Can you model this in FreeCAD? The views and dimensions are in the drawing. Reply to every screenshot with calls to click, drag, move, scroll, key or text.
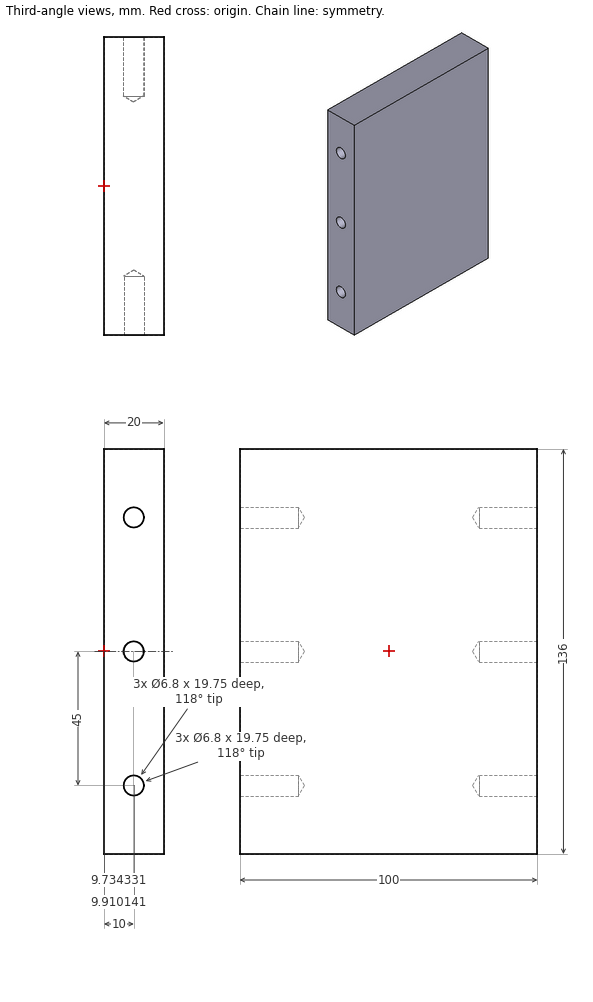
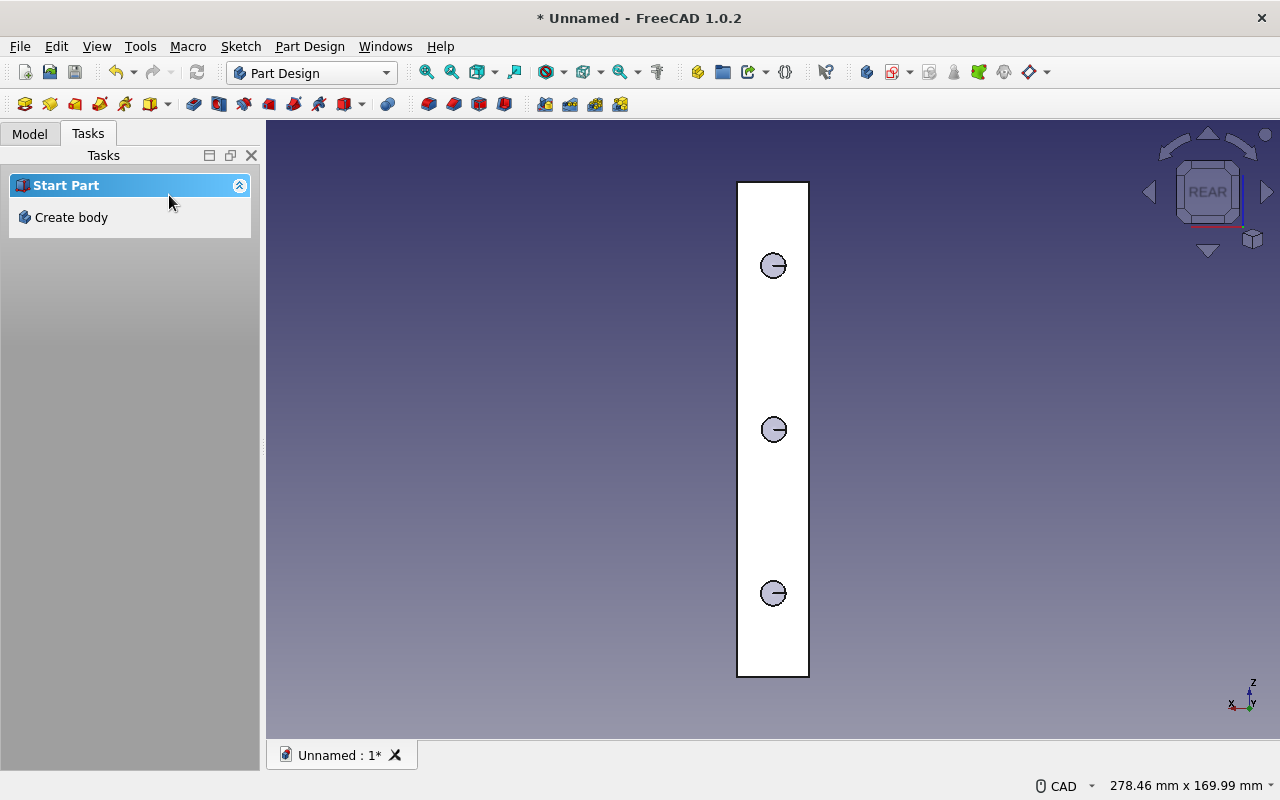
key(0)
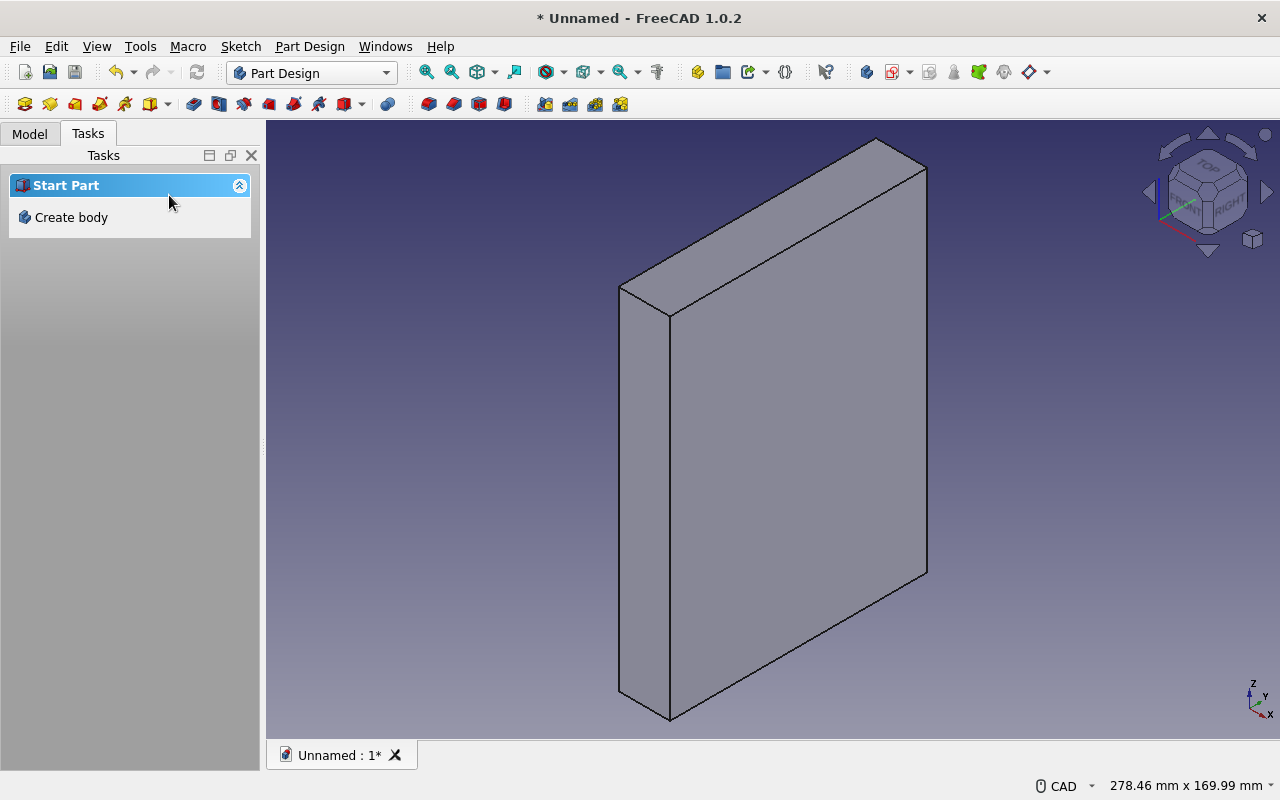
click(644, 503)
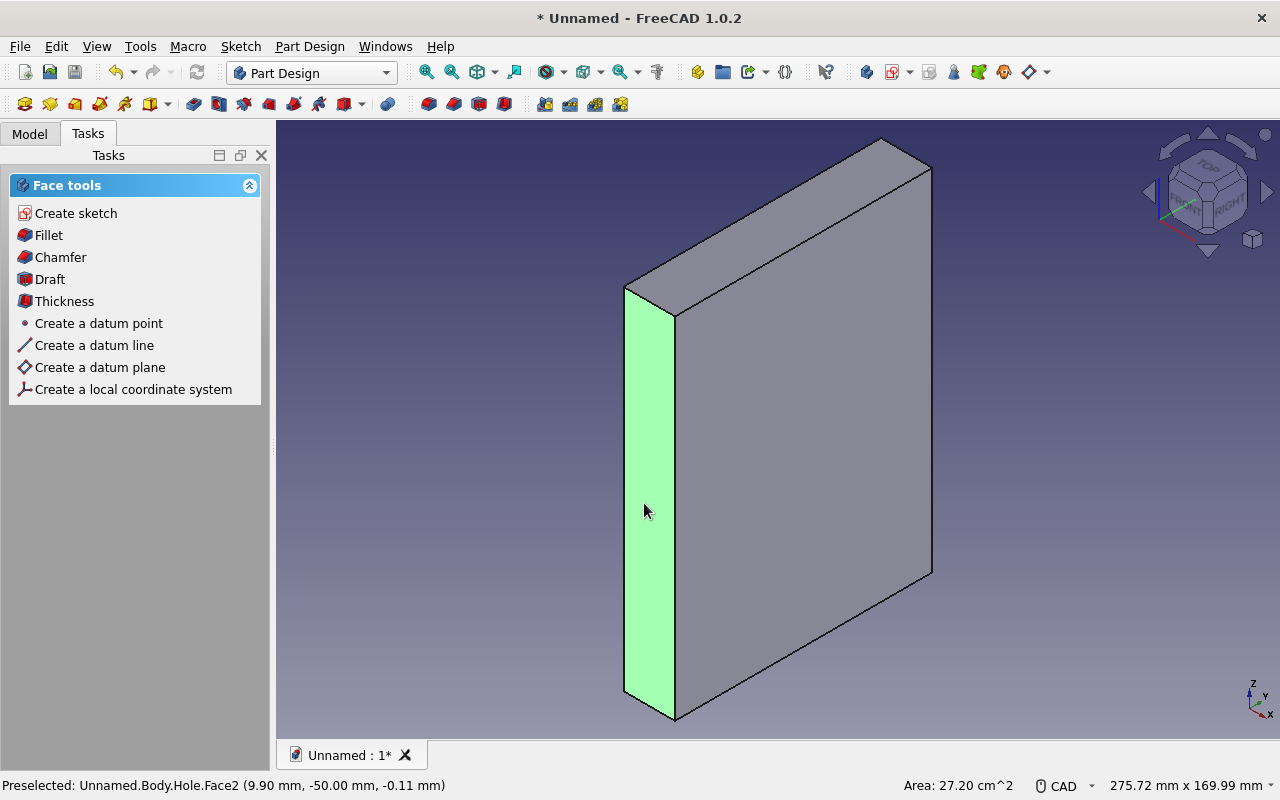
click(892, 72)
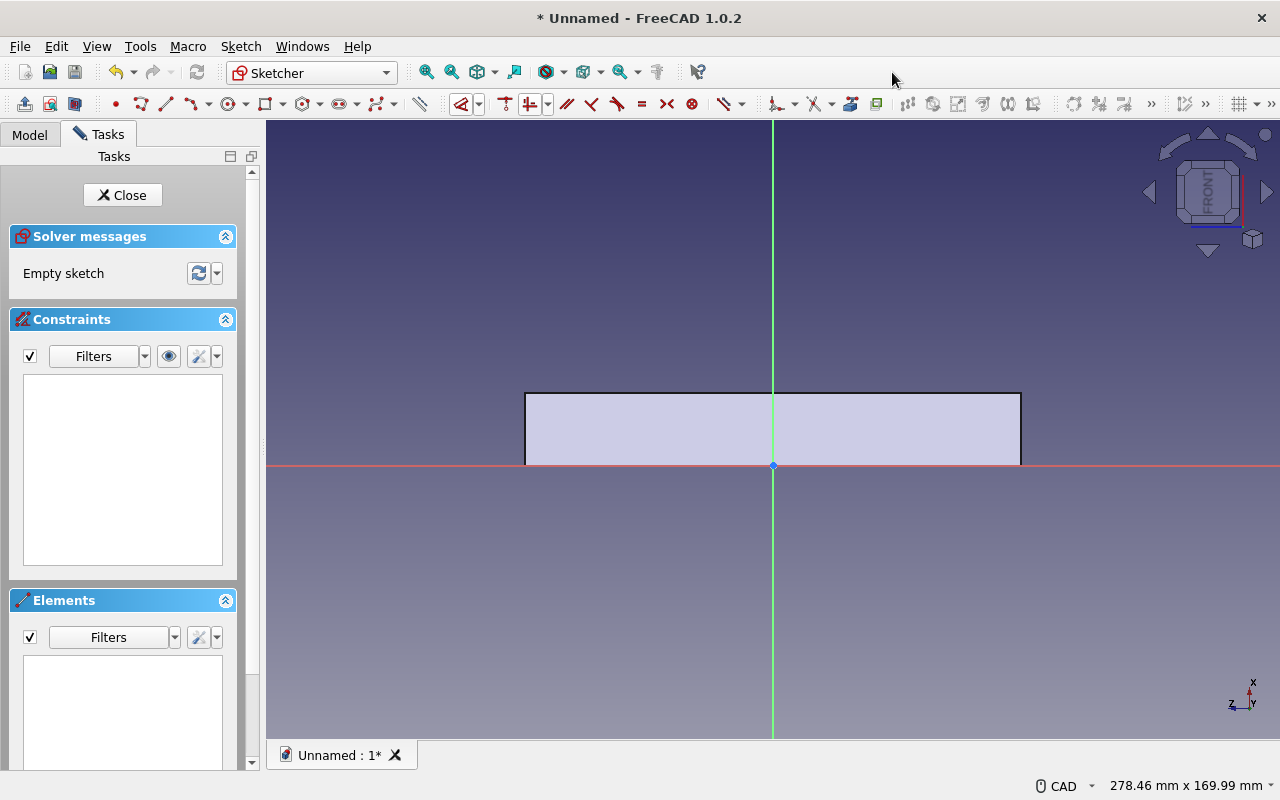
scroll(912, 466, up, 2)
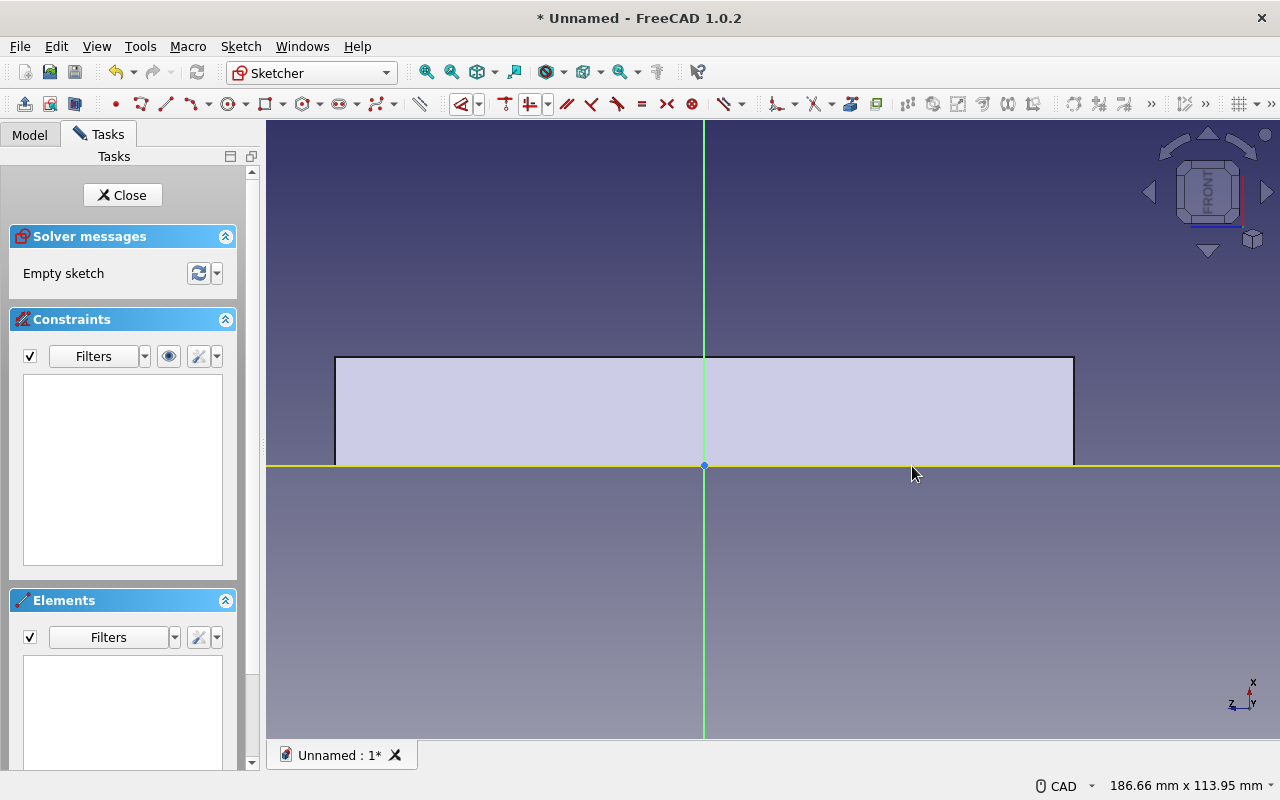
click(228, 104)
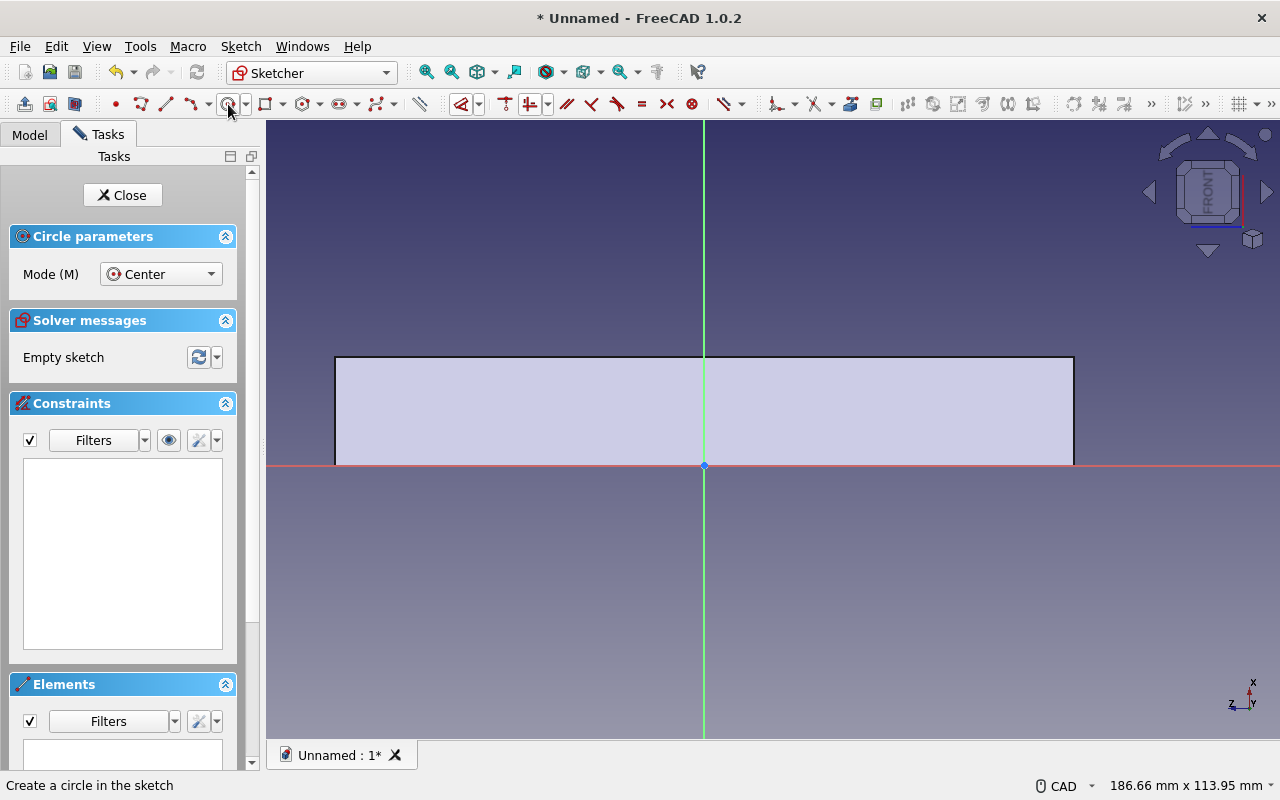
scroll(949, 411, up, 2)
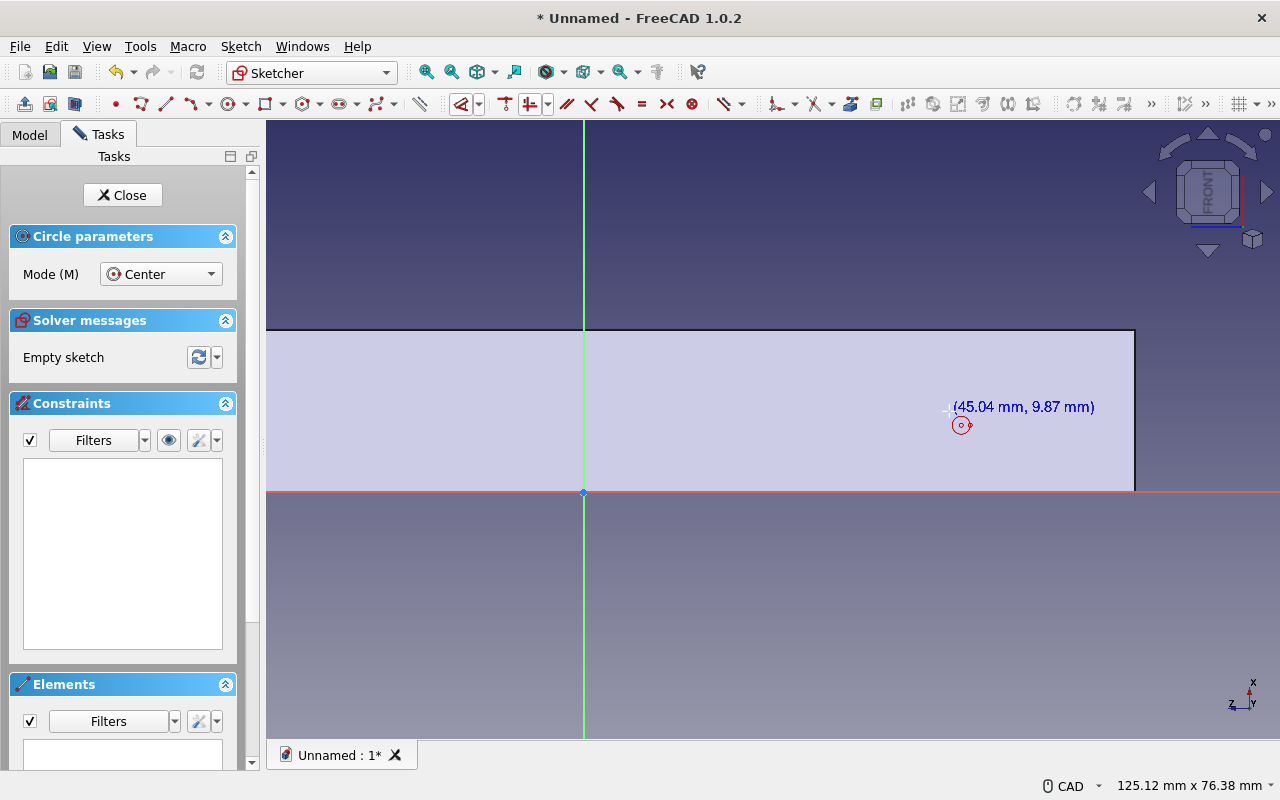
click(948, 411)
click(968, 392)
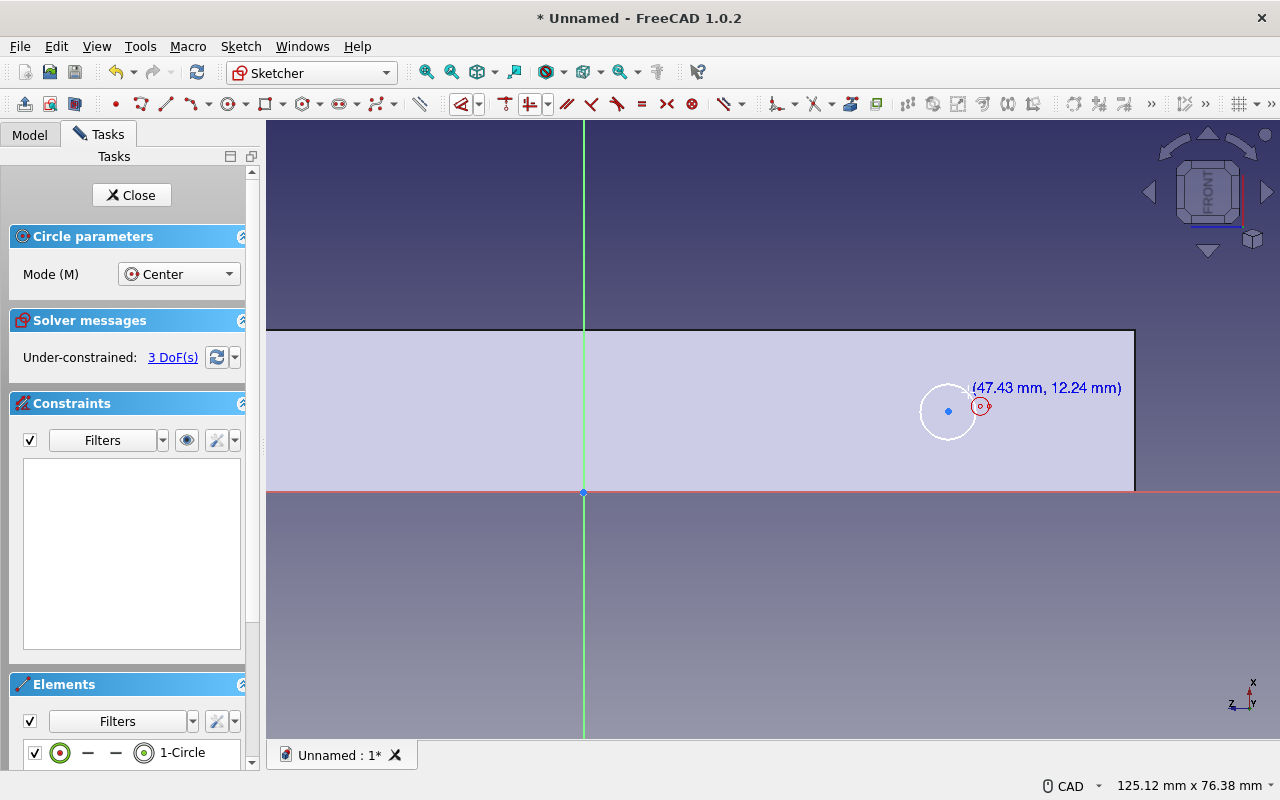
click(584, 411)
click(603, 392)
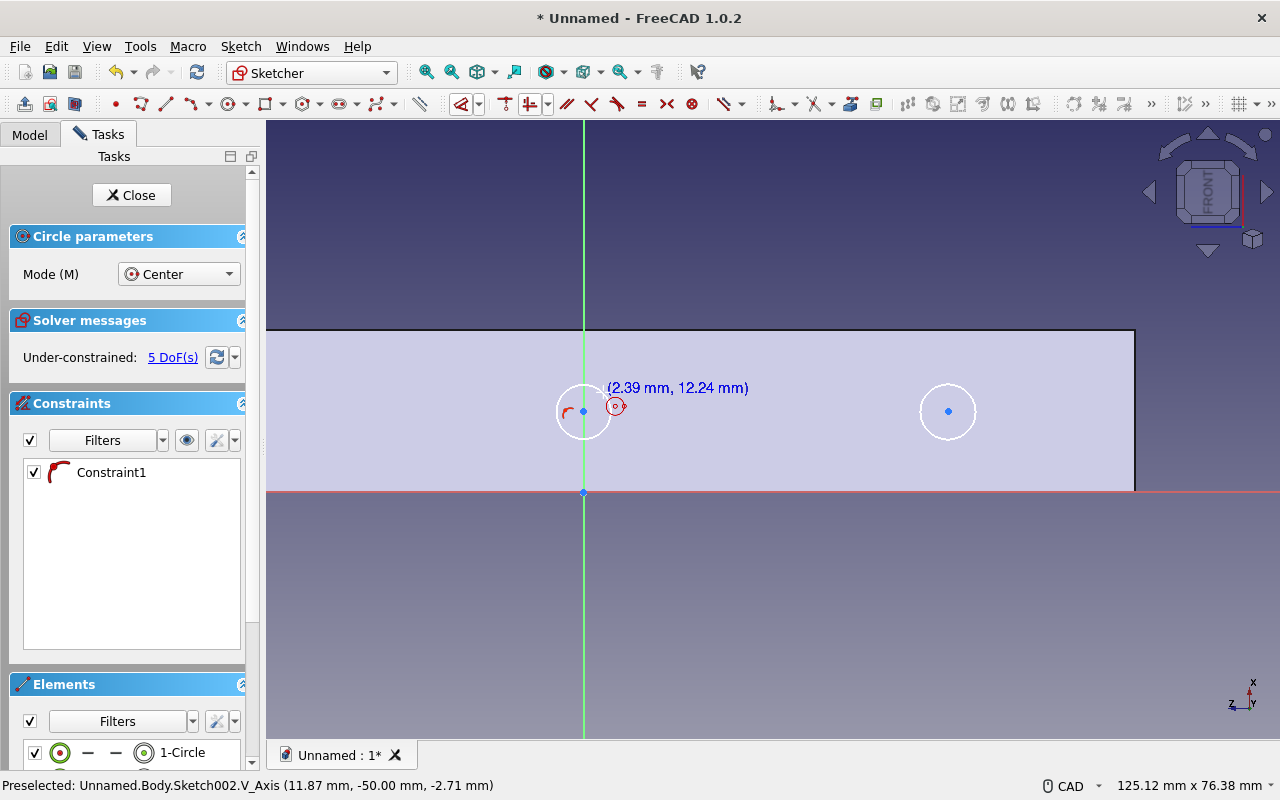
scroll(950, 412, down, 2)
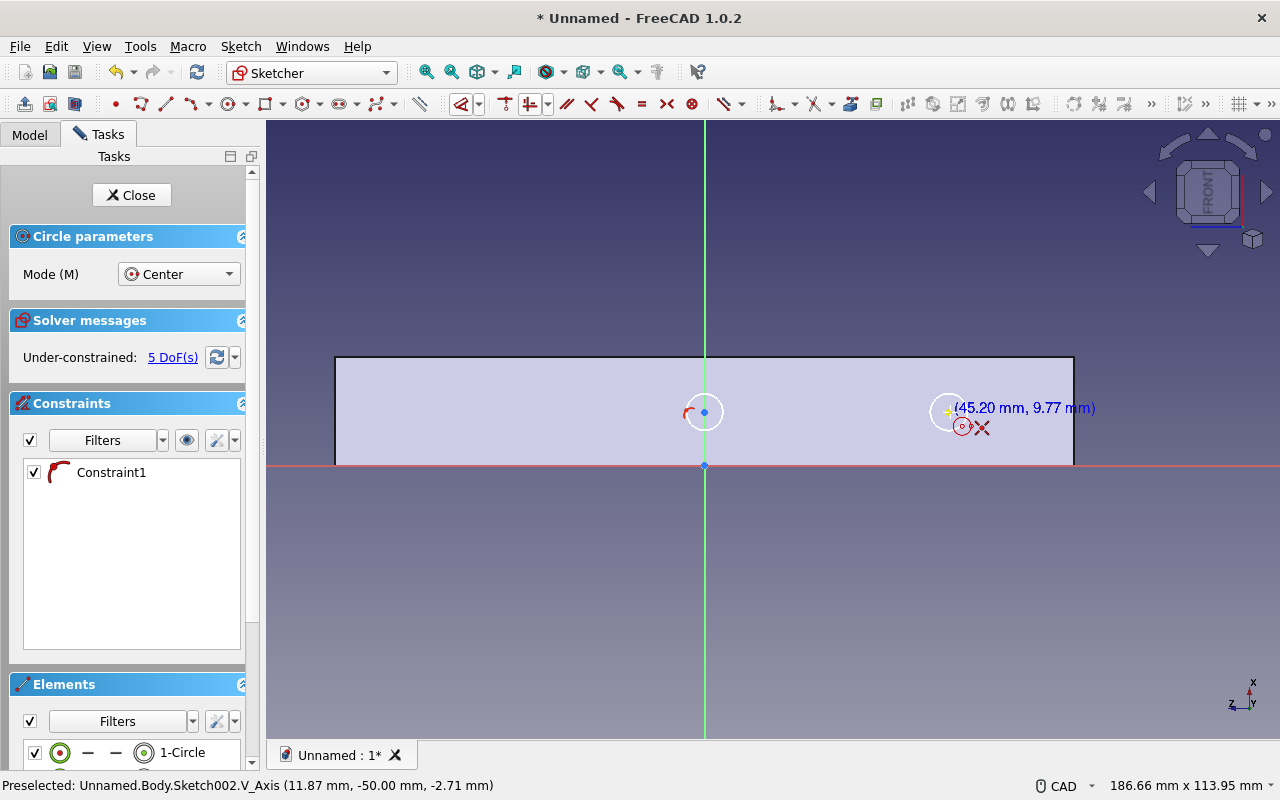
scroll(460, 412, up, 2)